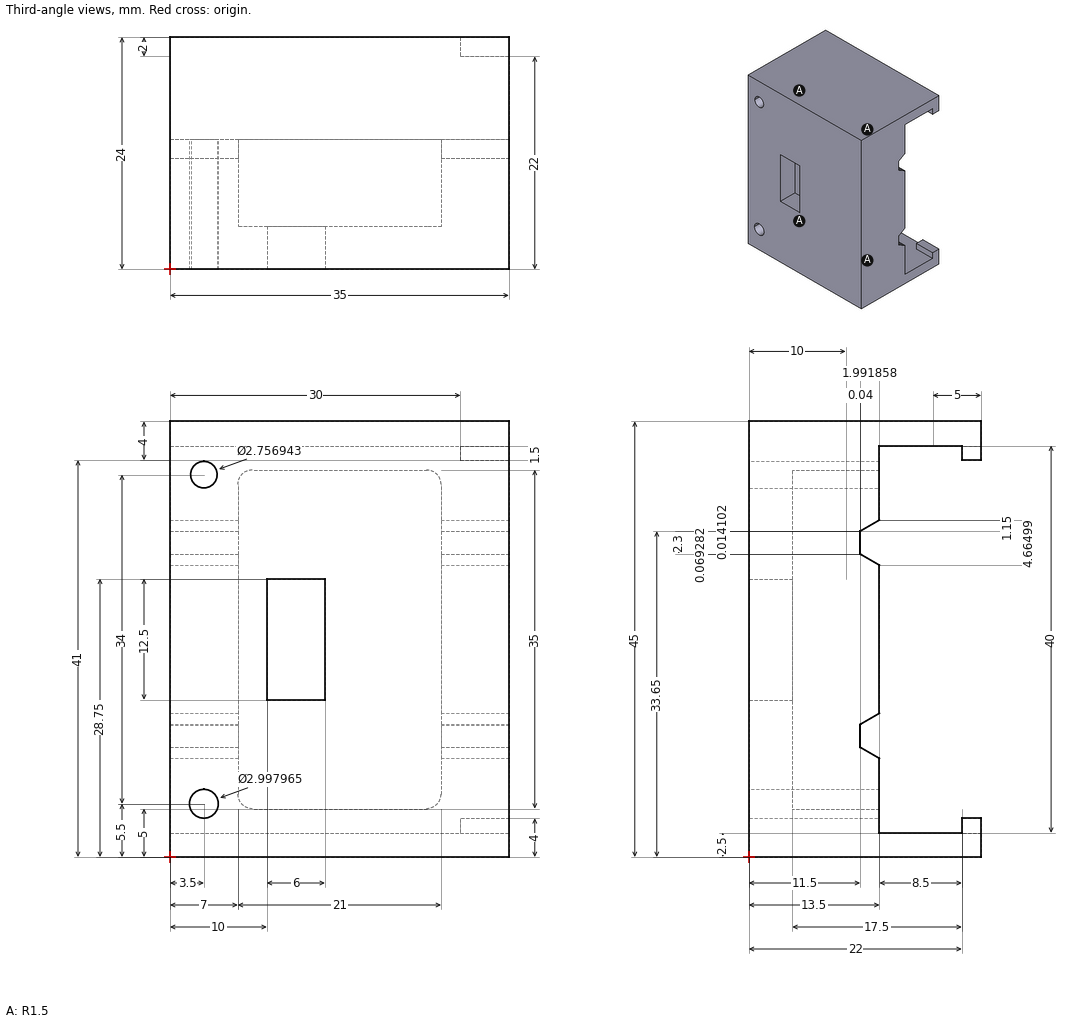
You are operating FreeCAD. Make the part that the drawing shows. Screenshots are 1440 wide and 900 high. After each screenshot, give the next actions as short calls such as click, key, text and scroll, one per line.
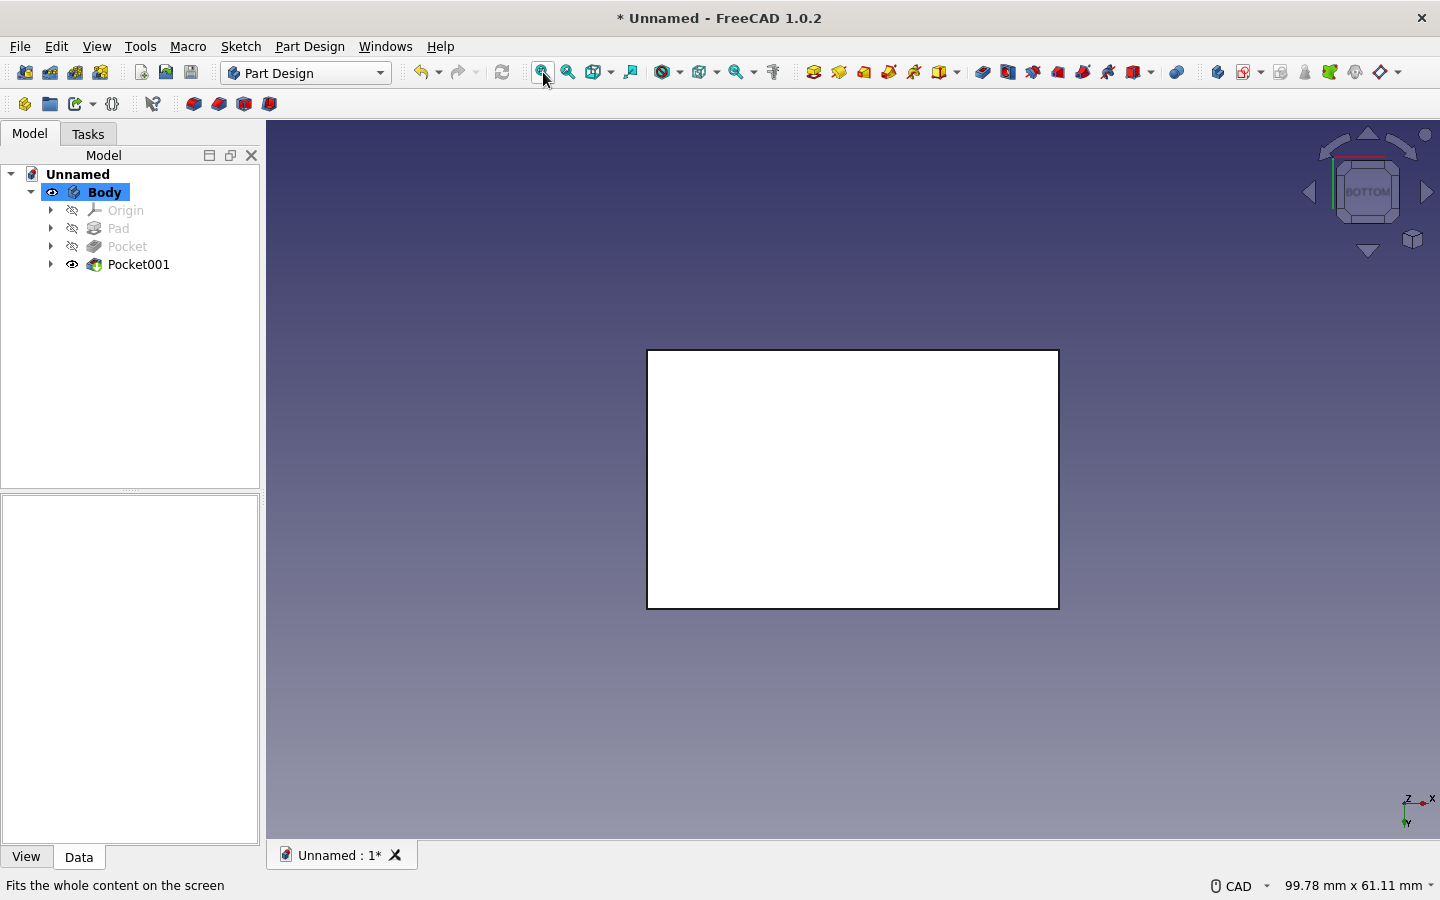
click(543, 72)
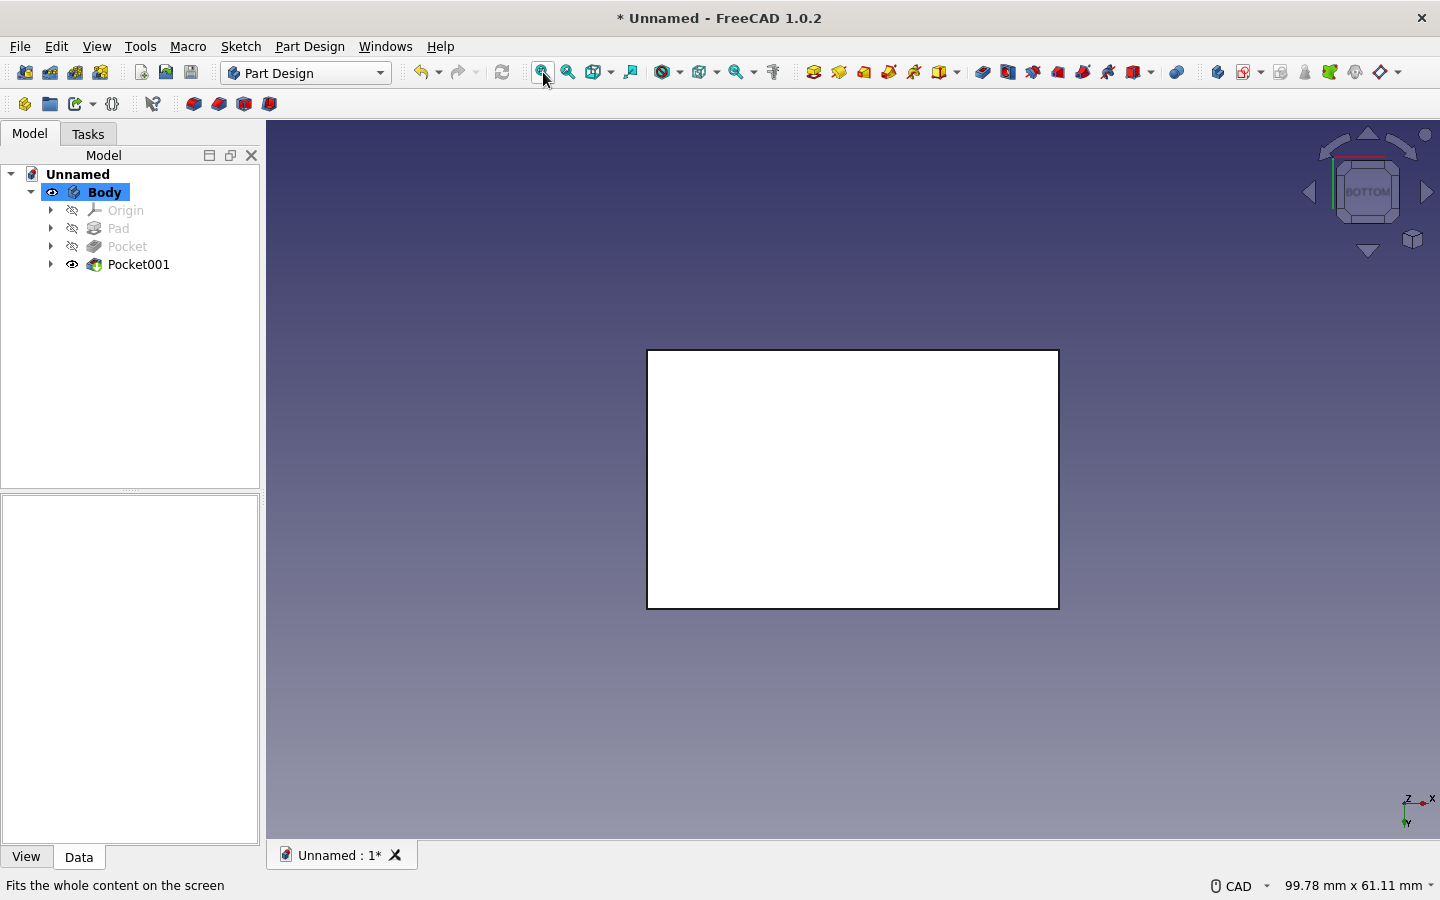
key(4)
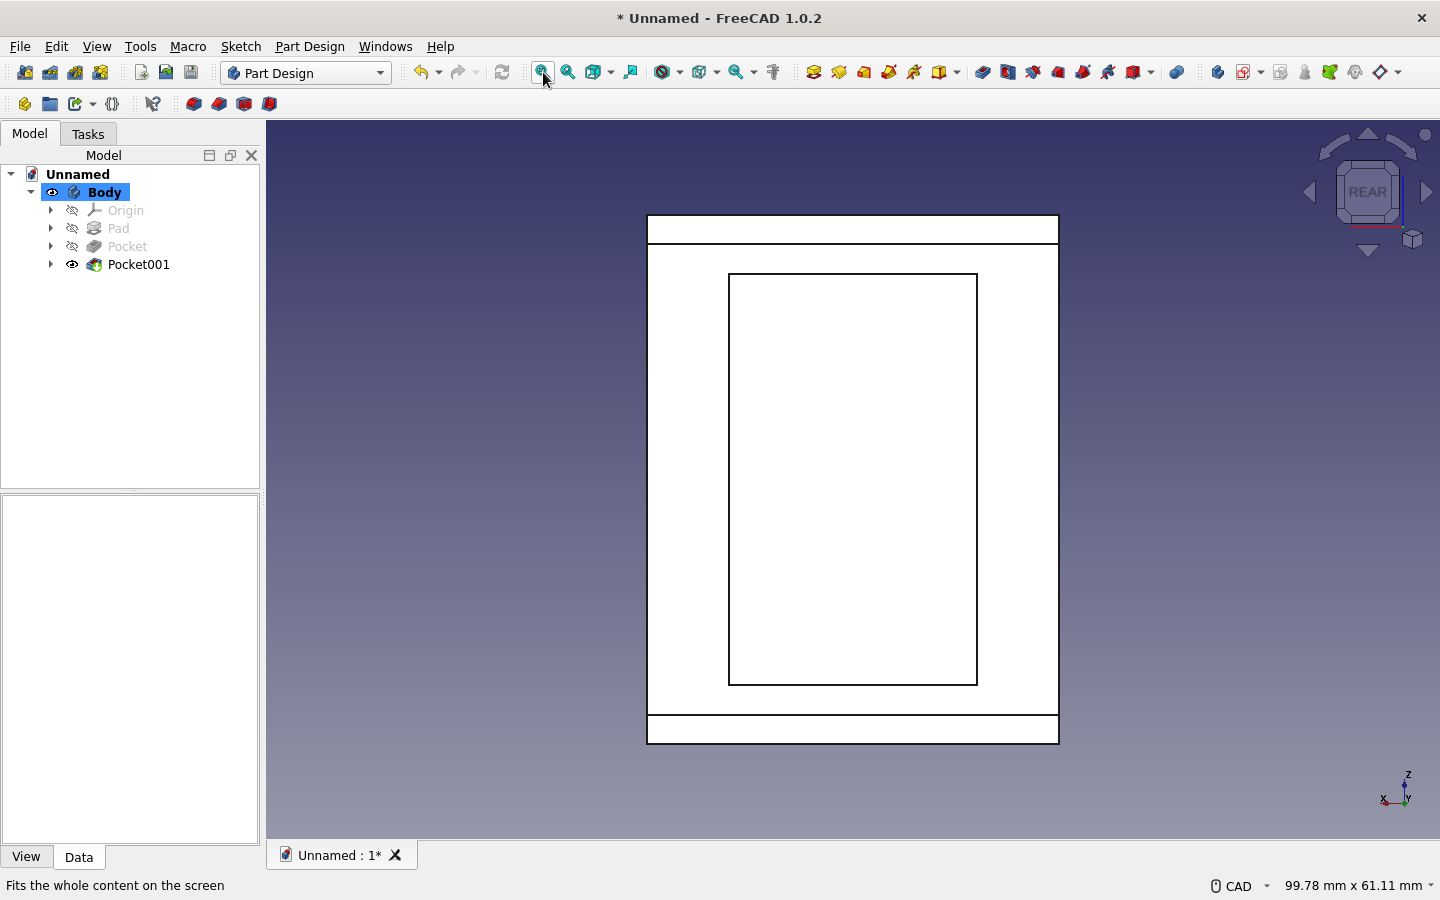
key(6)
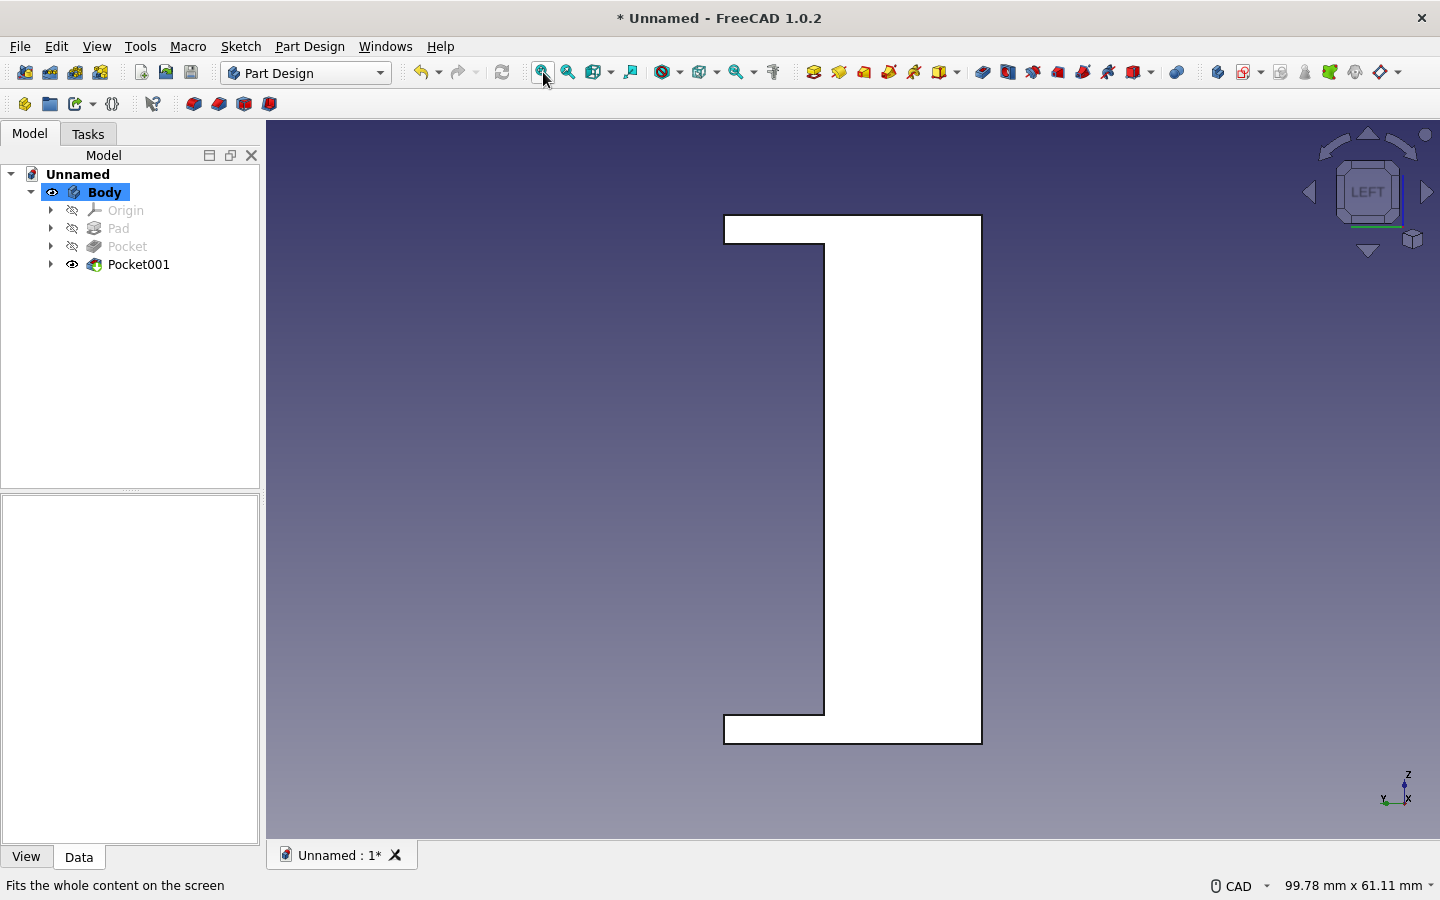
key(v)
key(3)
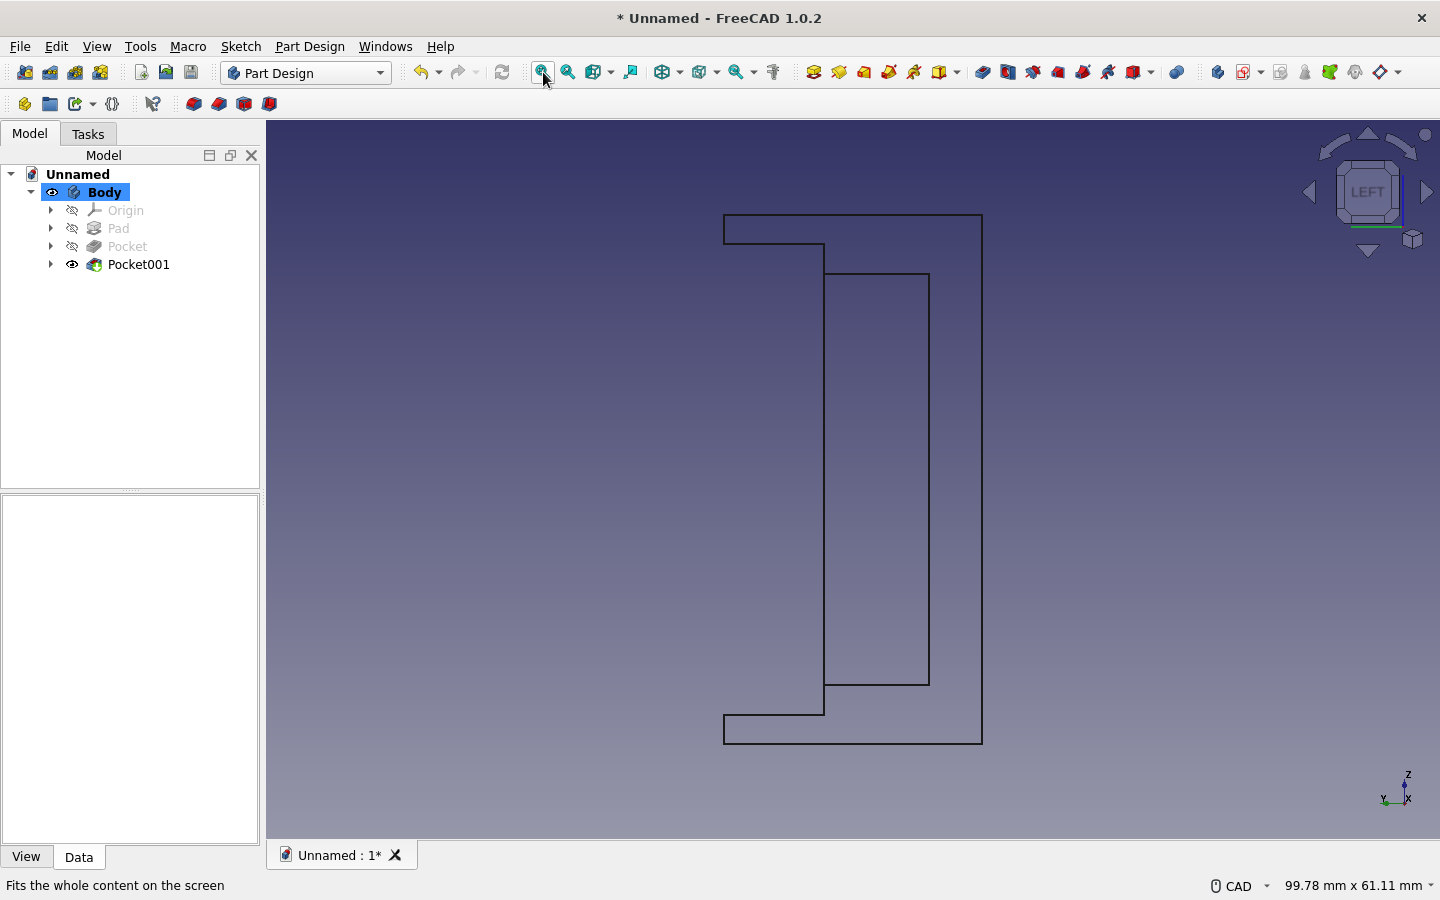
key(0)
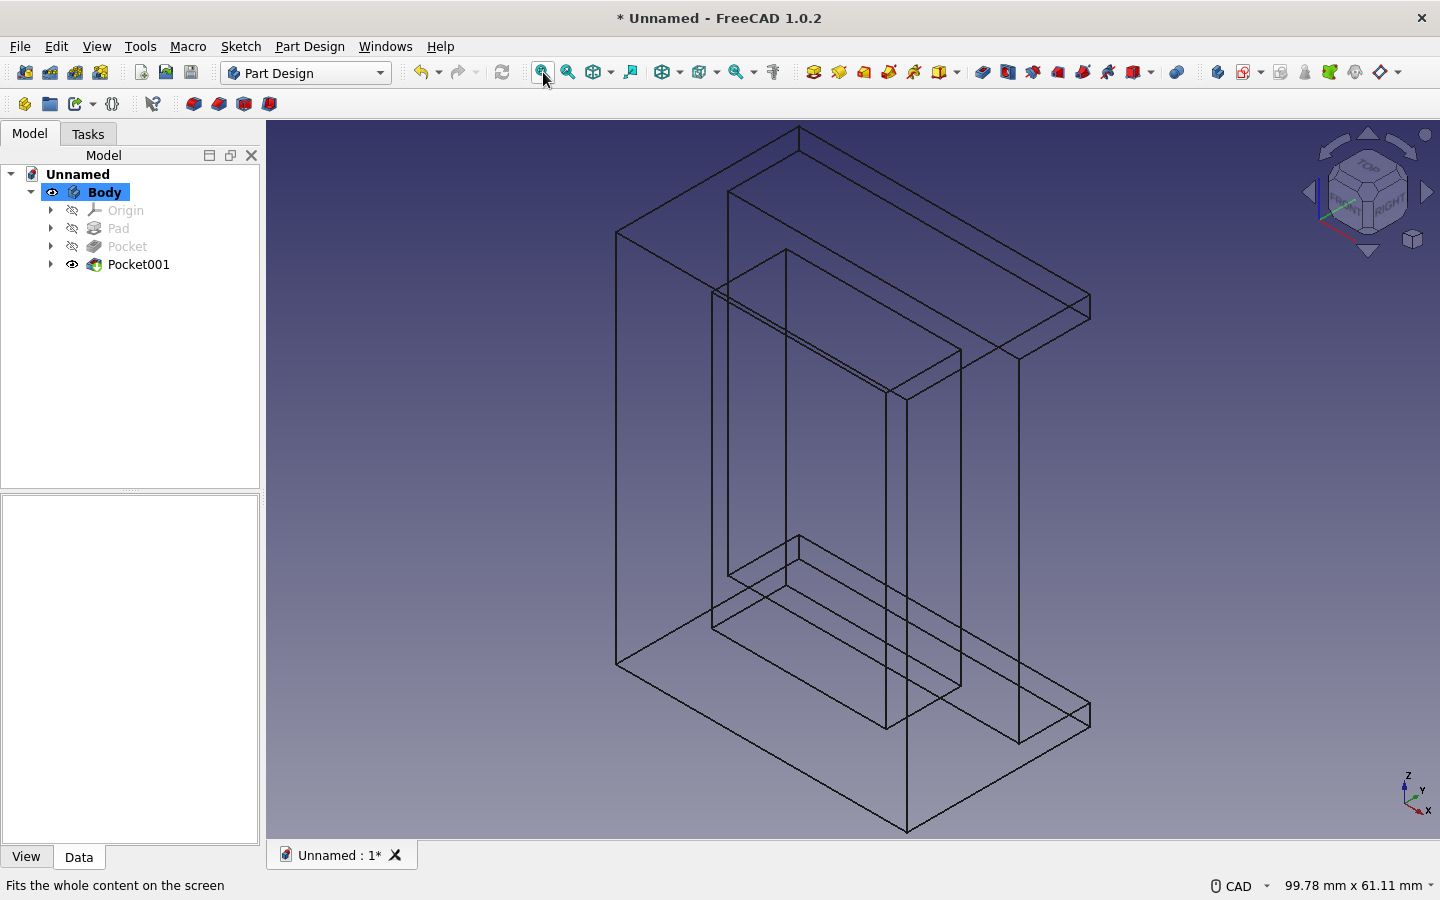
click(749, 606)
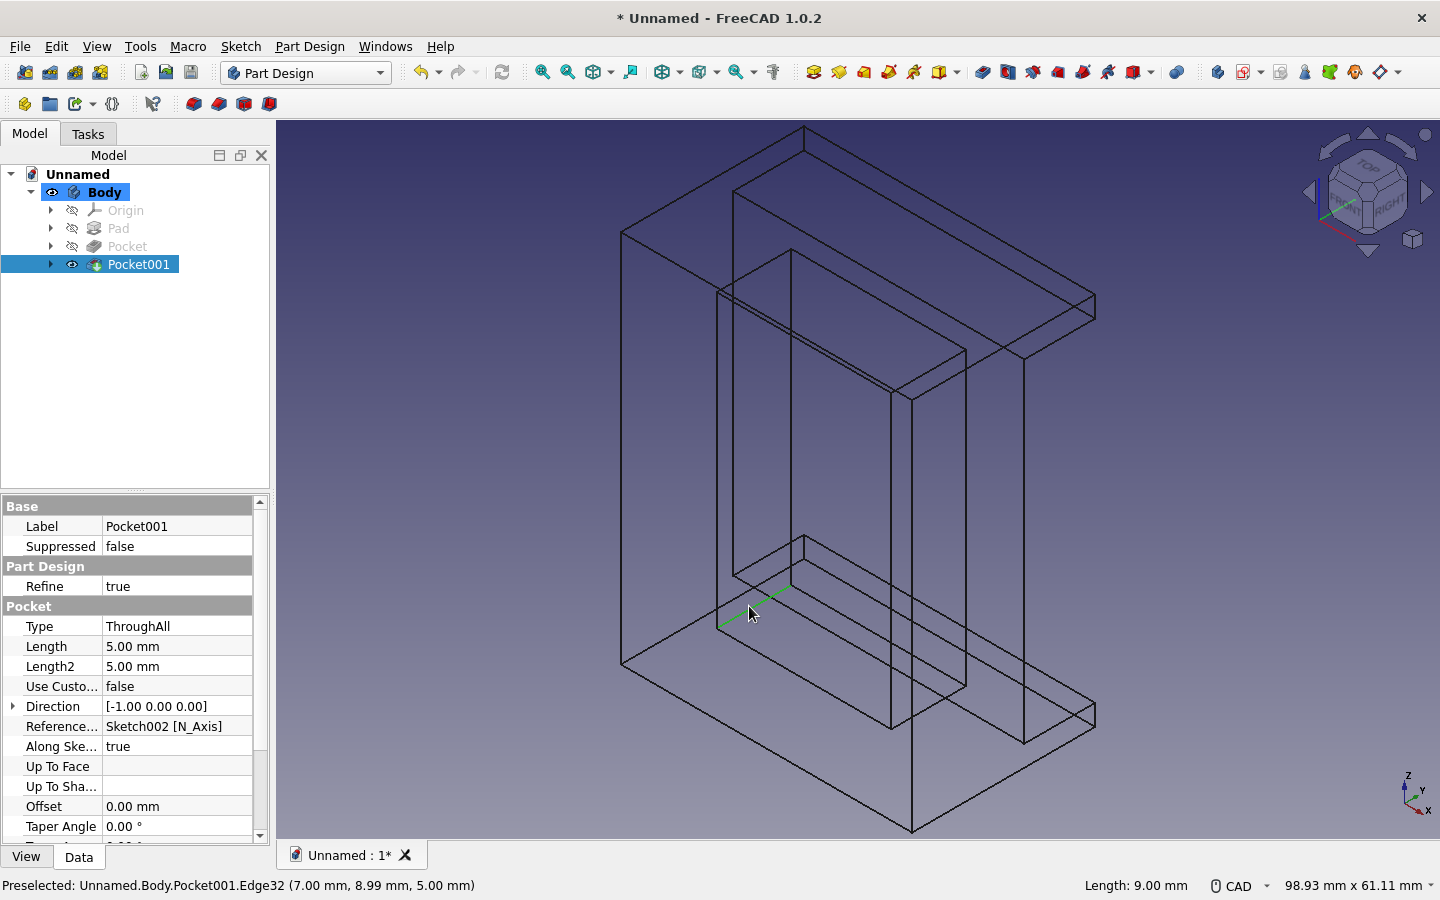
click(929, 707, ctrl)